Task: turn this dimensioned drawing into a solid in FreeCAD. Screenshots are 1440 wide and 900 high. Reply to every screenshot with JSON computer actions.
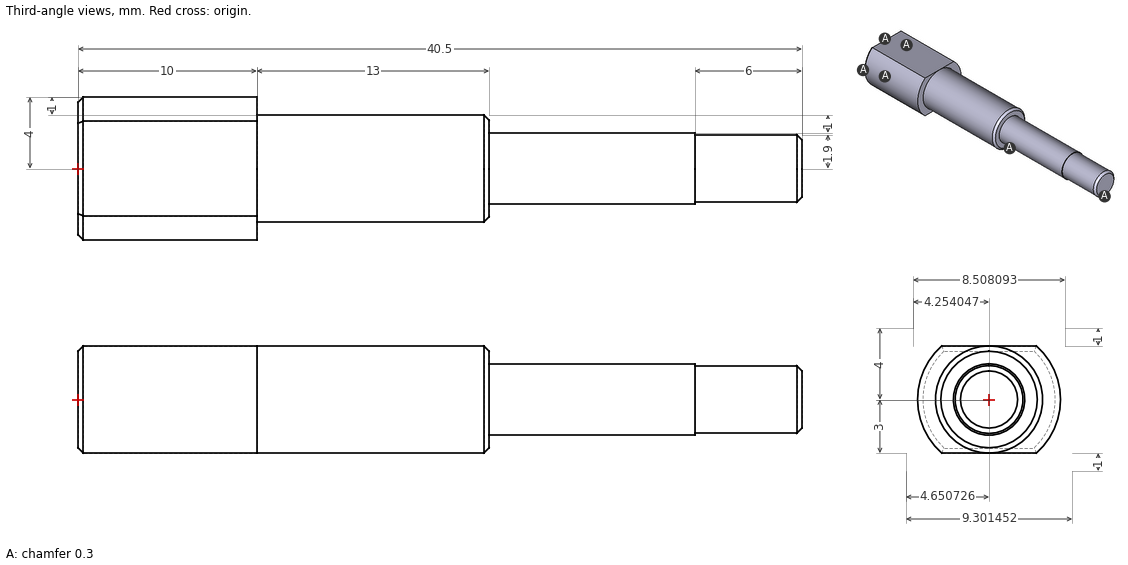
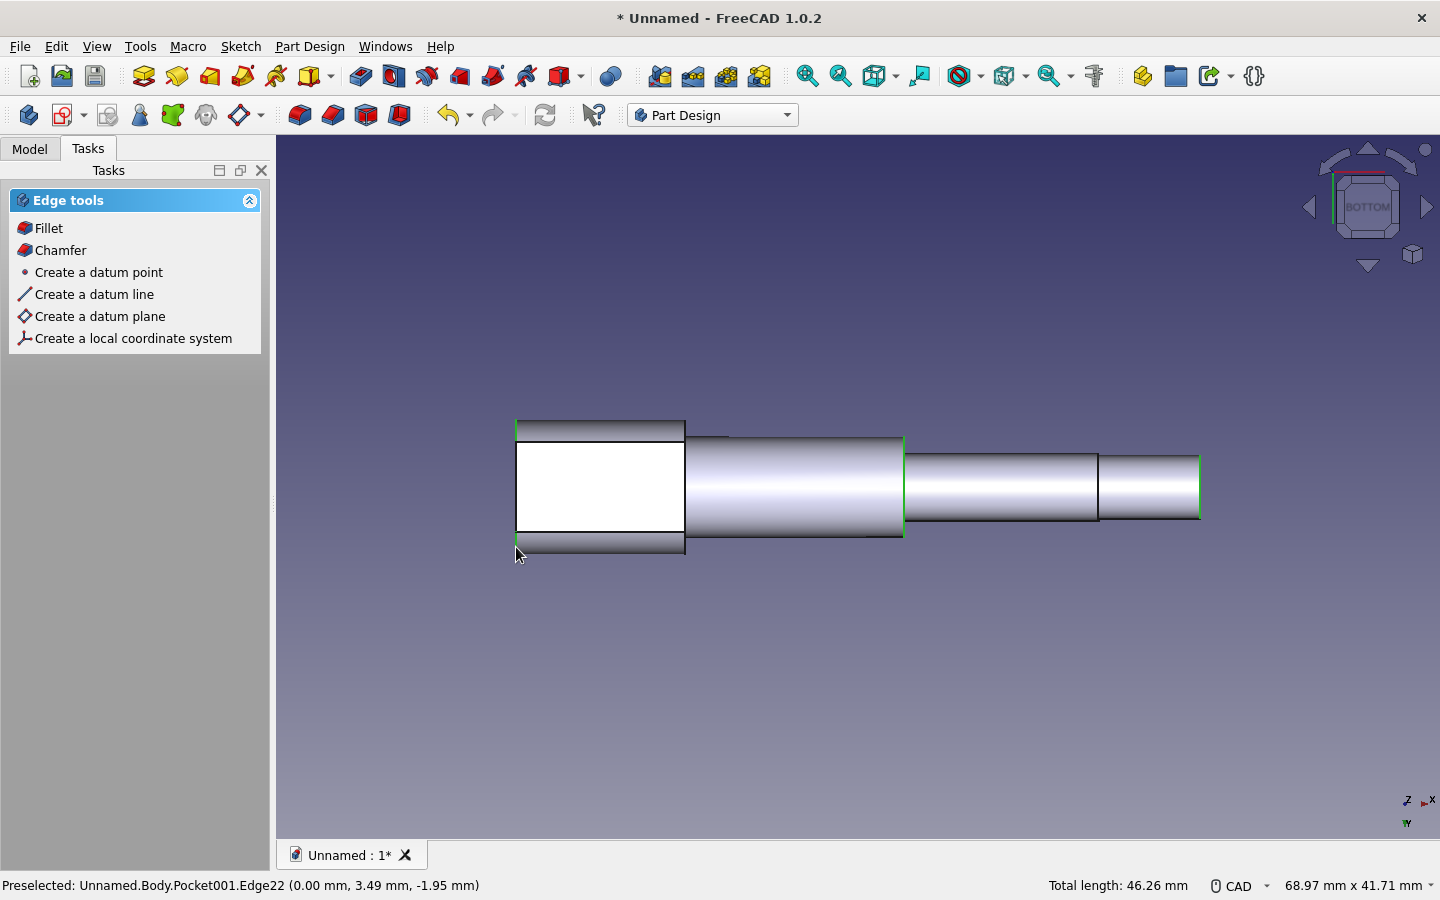
{"action": "left_click", "coordinate": [516, 486], "text": "ctrl"}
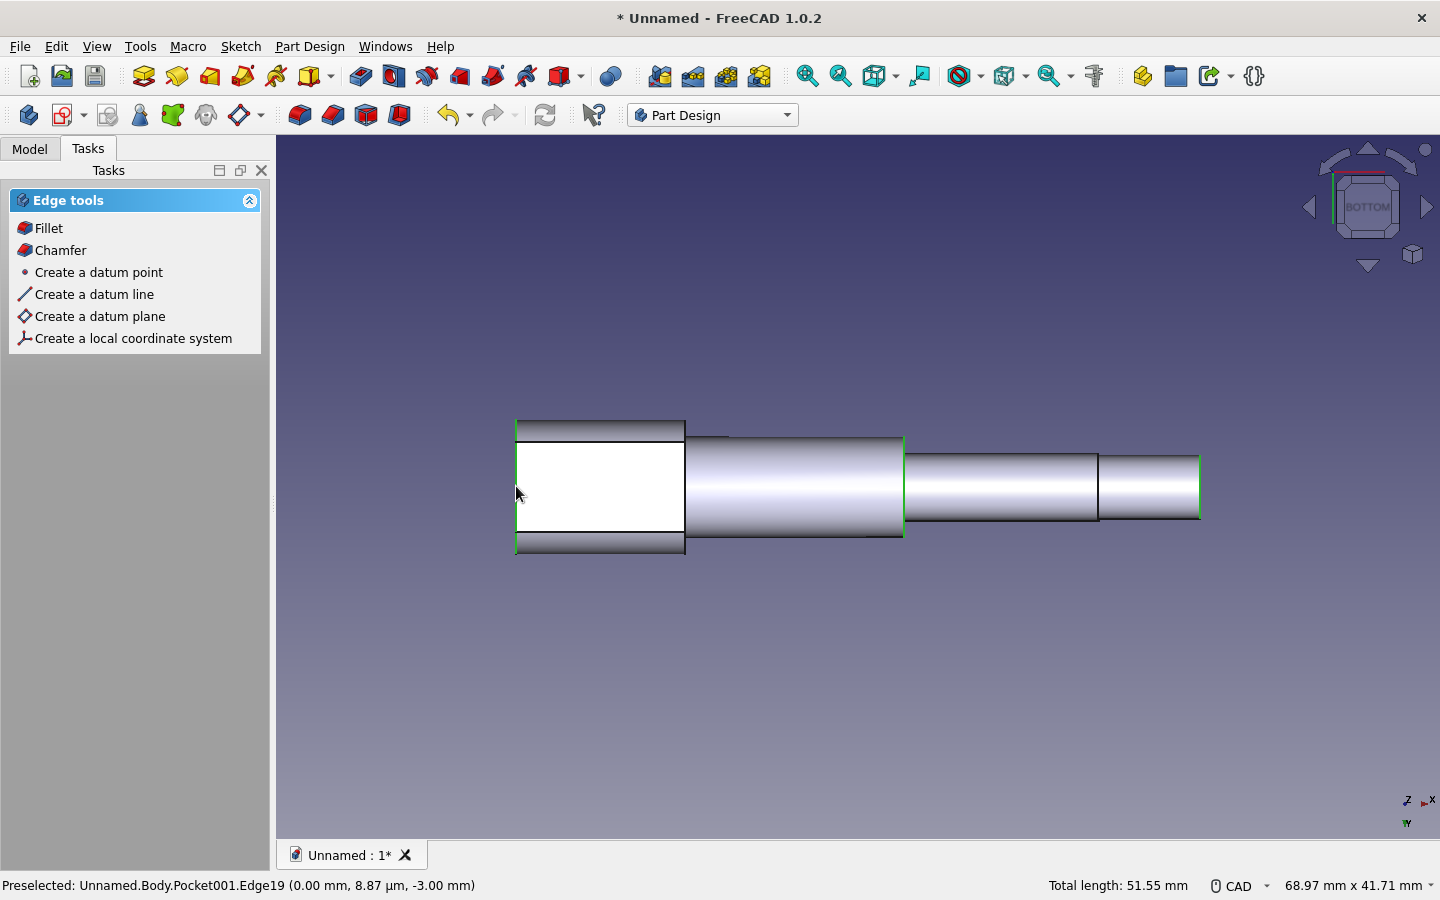
{"action": "left_click", "coordinate": [333, 116]}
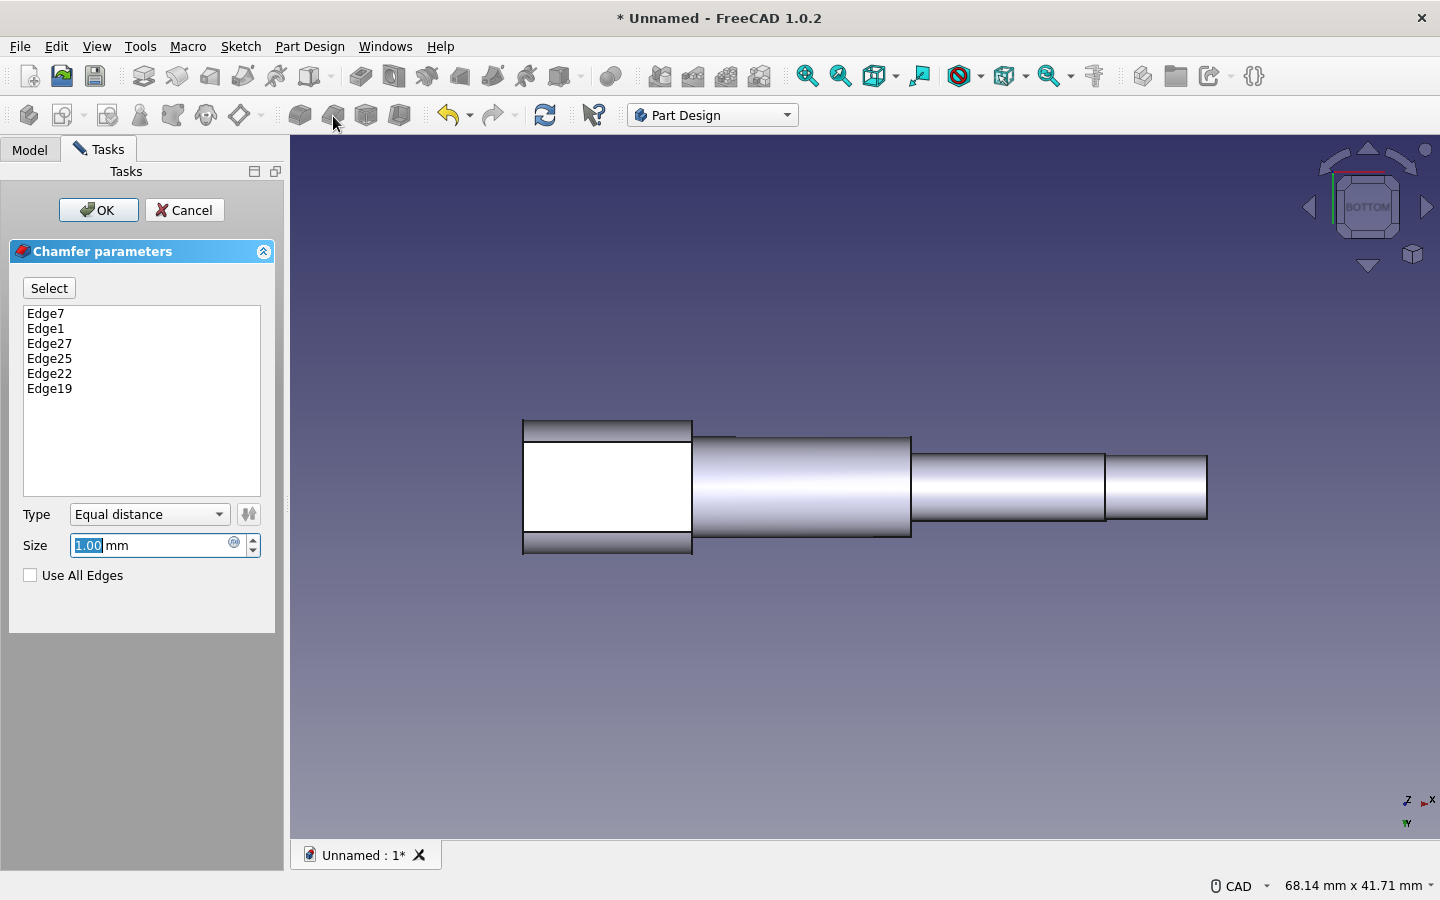
{"action": "type", "text": "0.3"}
{"action": "key", "text": "Tab"}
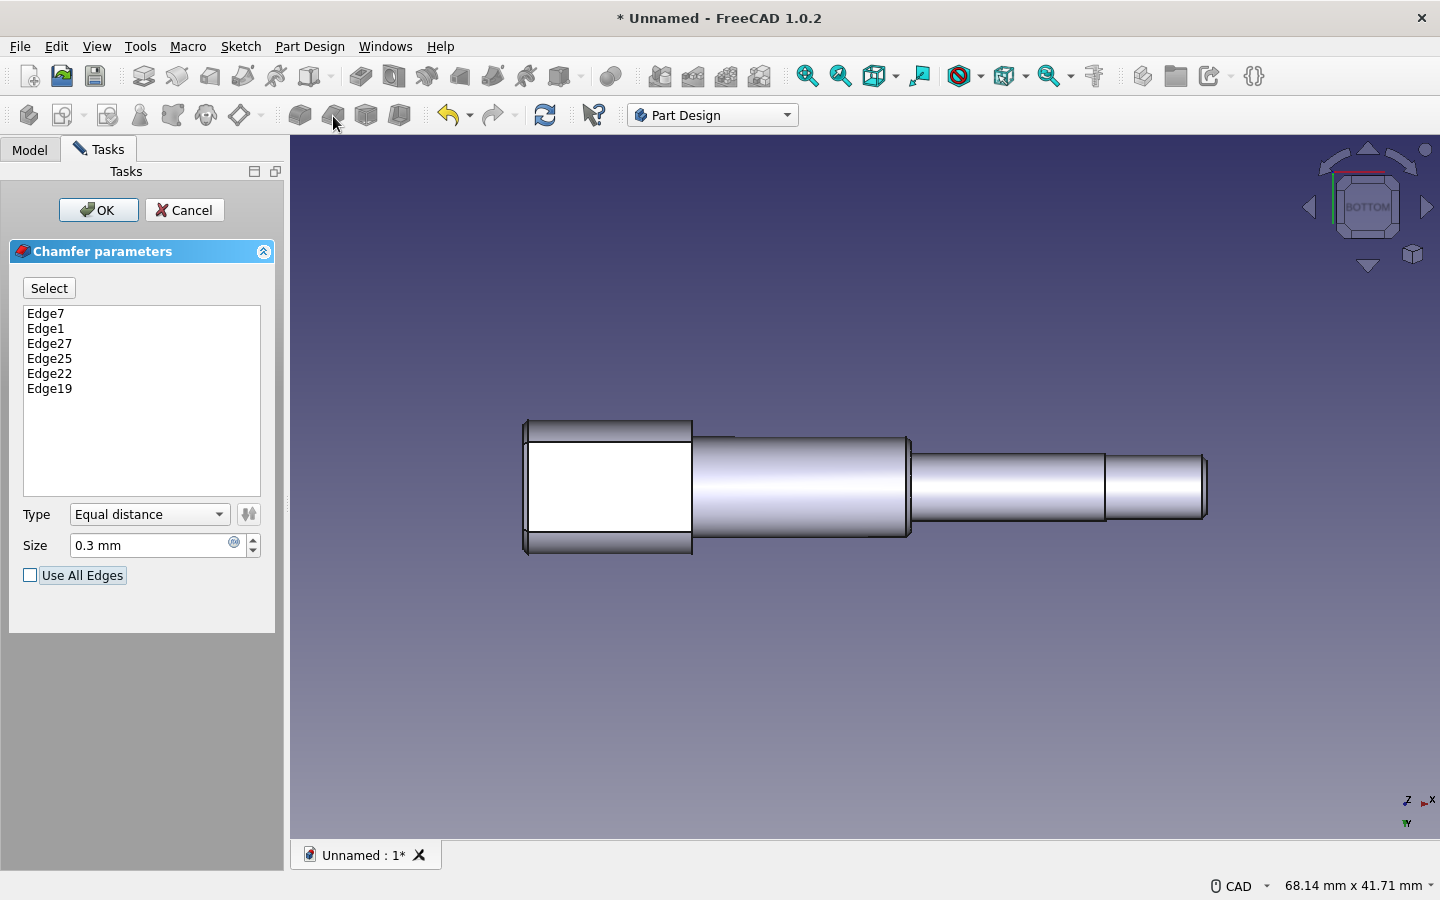
{"action": "left_click", "coordinate": [99, 210]}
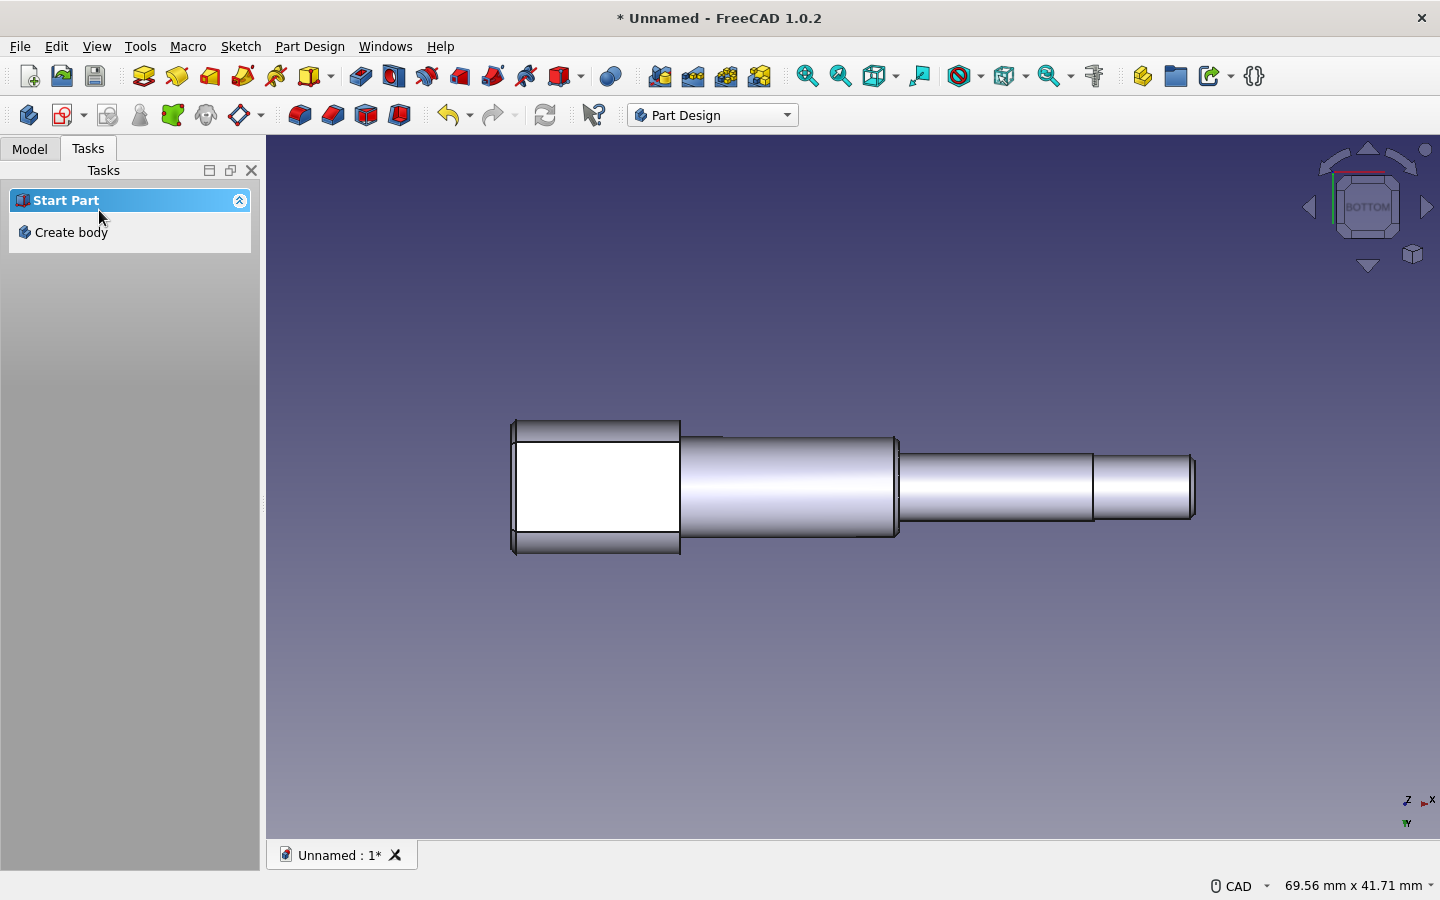
{"action": "key", "text": "0"}